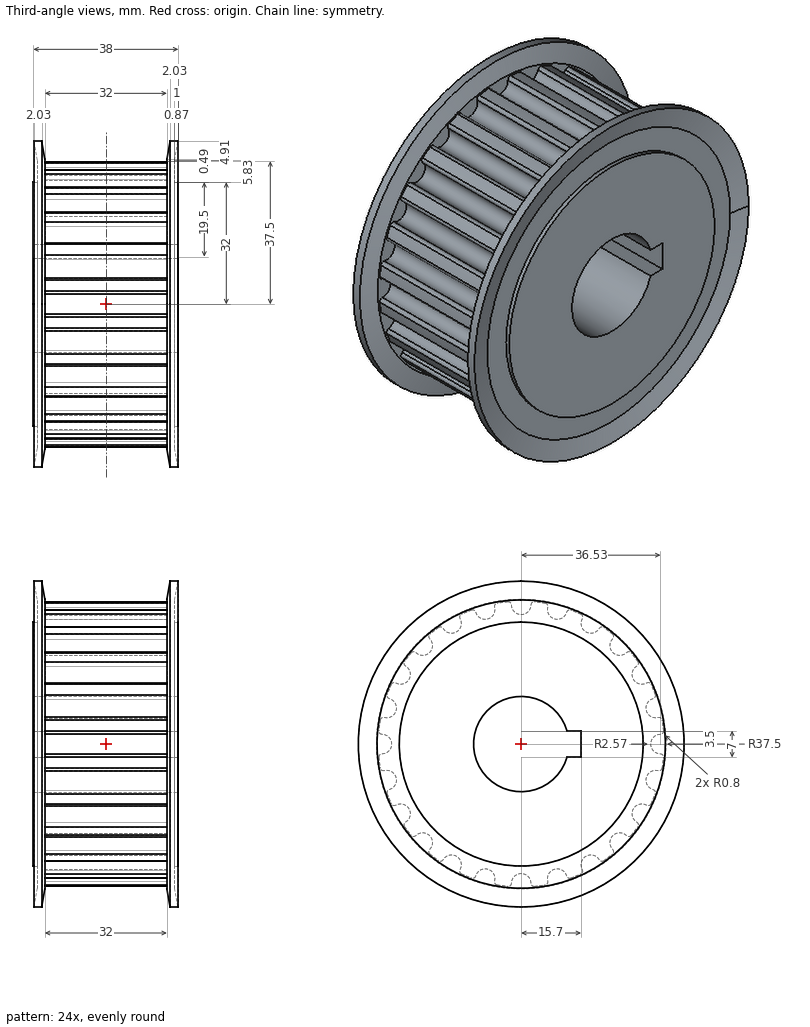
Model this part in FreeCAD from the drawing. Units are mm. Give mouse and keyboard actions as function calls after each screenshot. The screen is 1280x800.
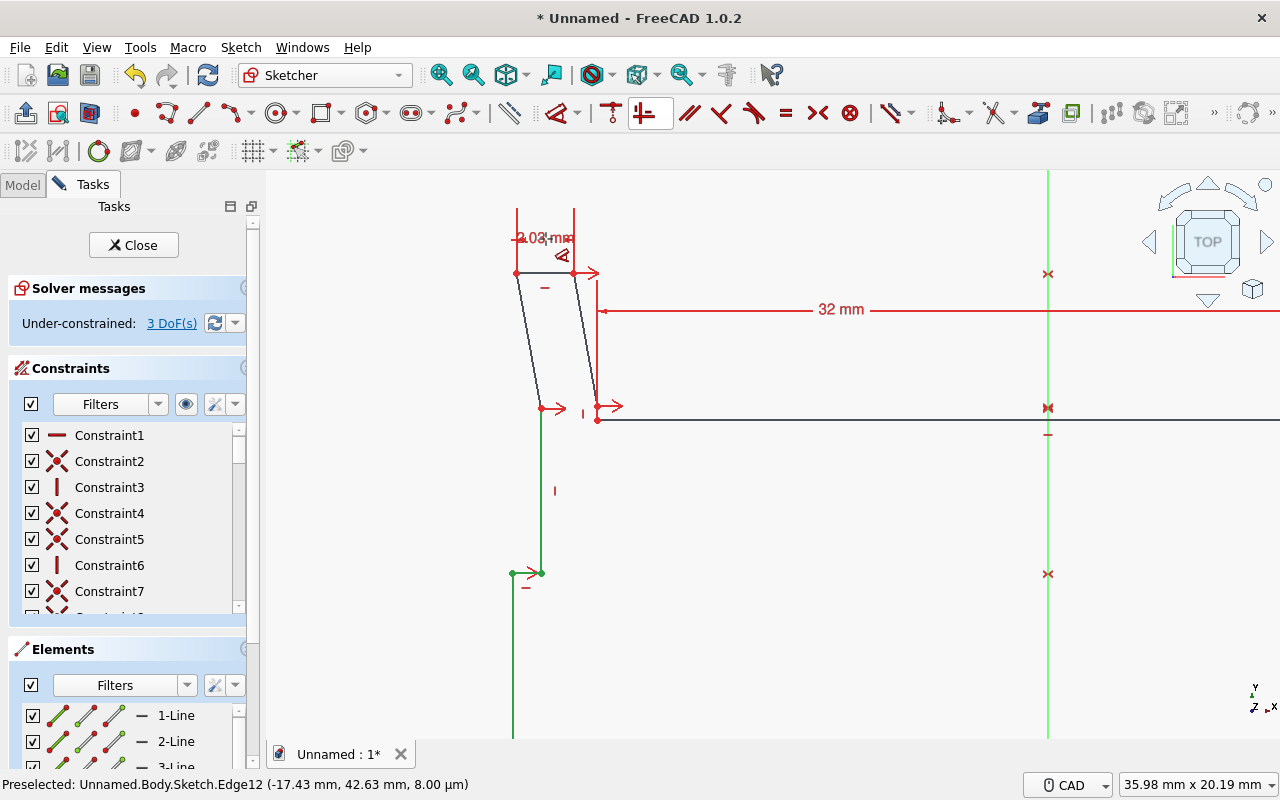
scroll(556, 274, down, 6)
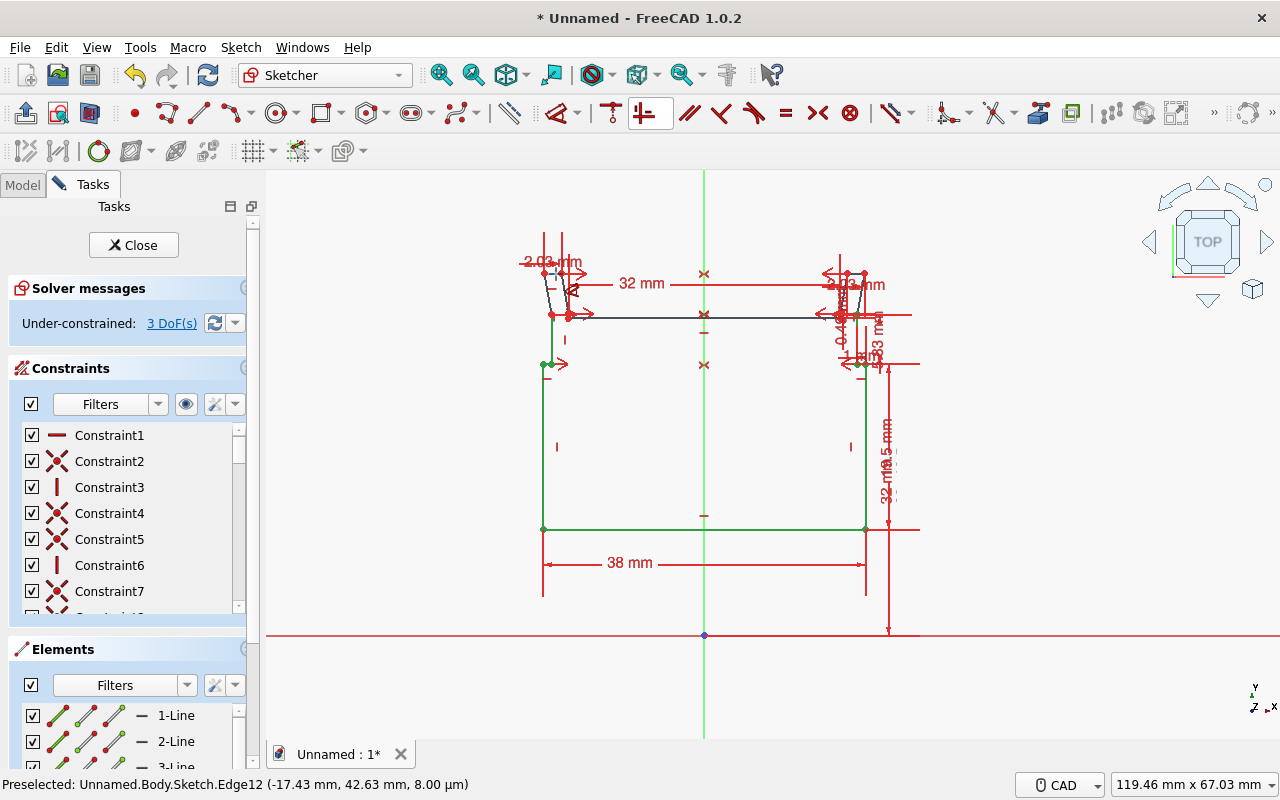
scroll(840, 318, up, 6)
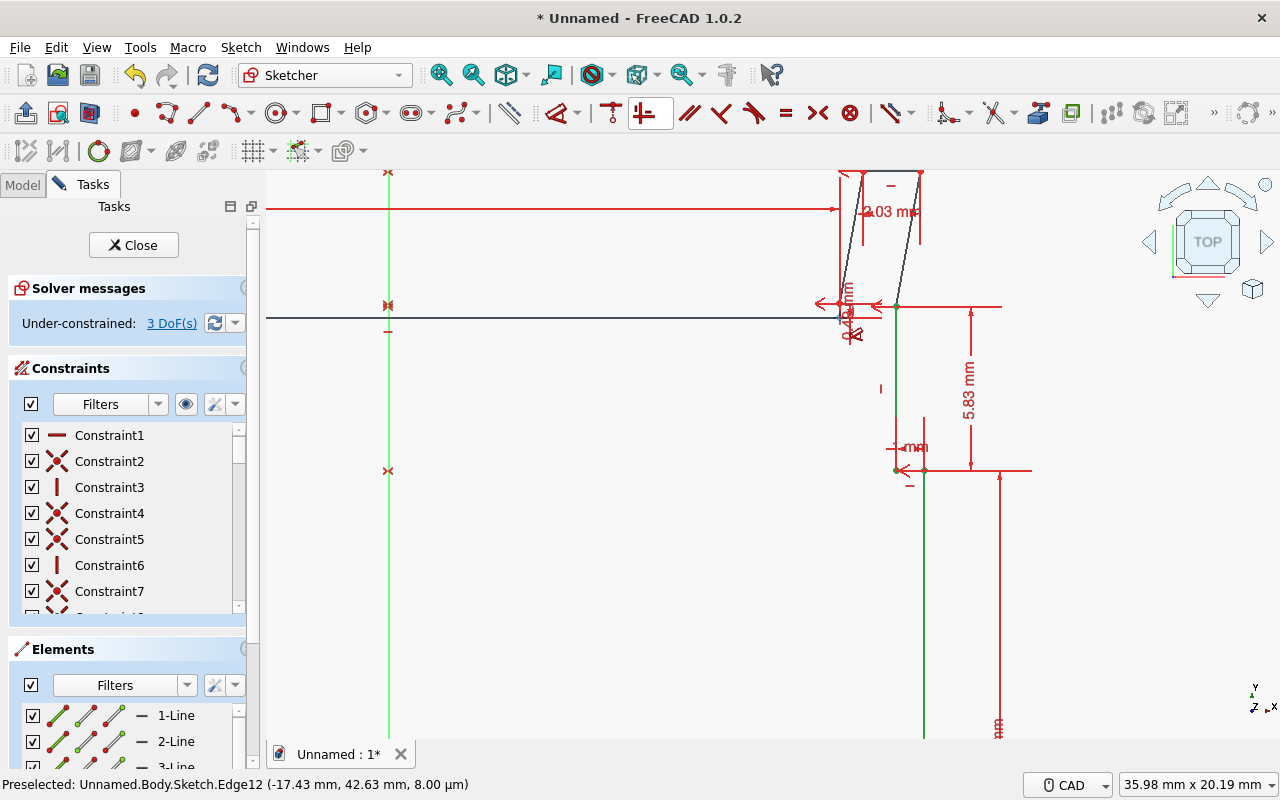
click(840, 318)
click(874, 514)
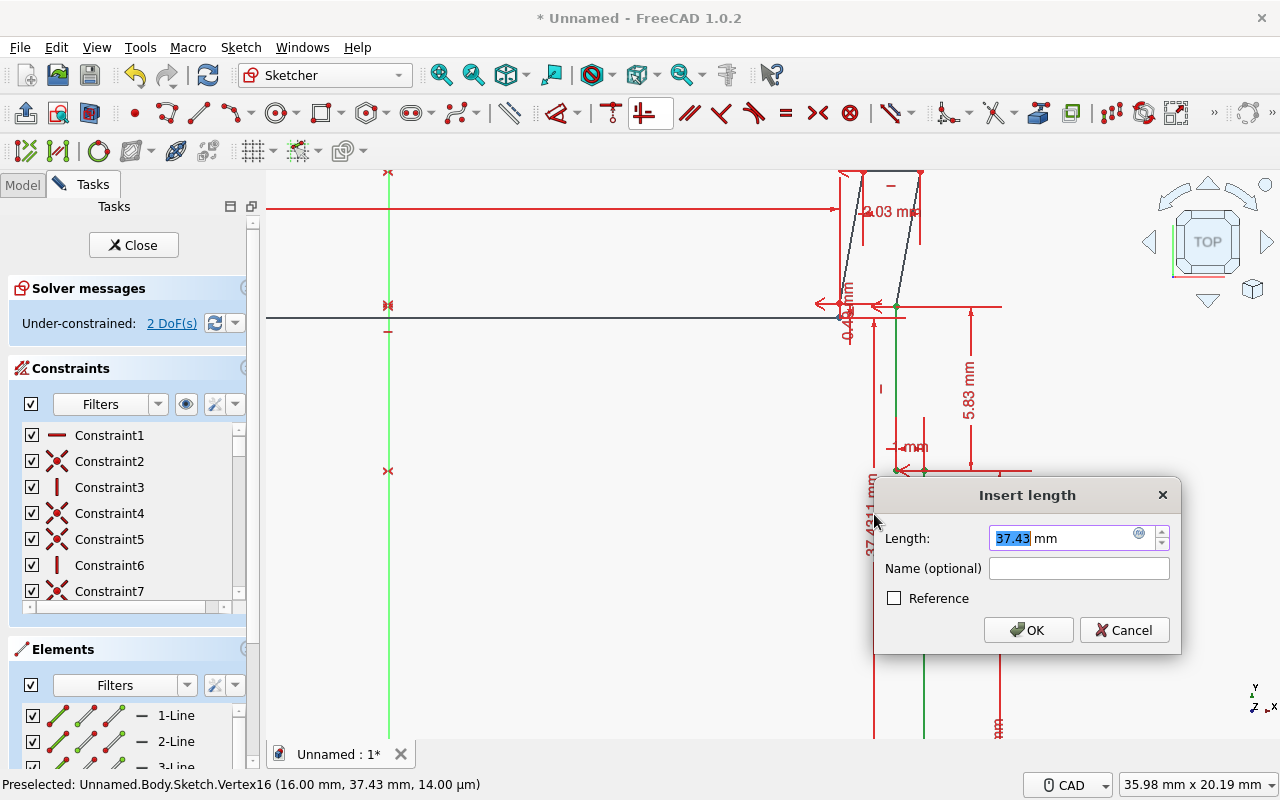
text(37.5)
key(Return)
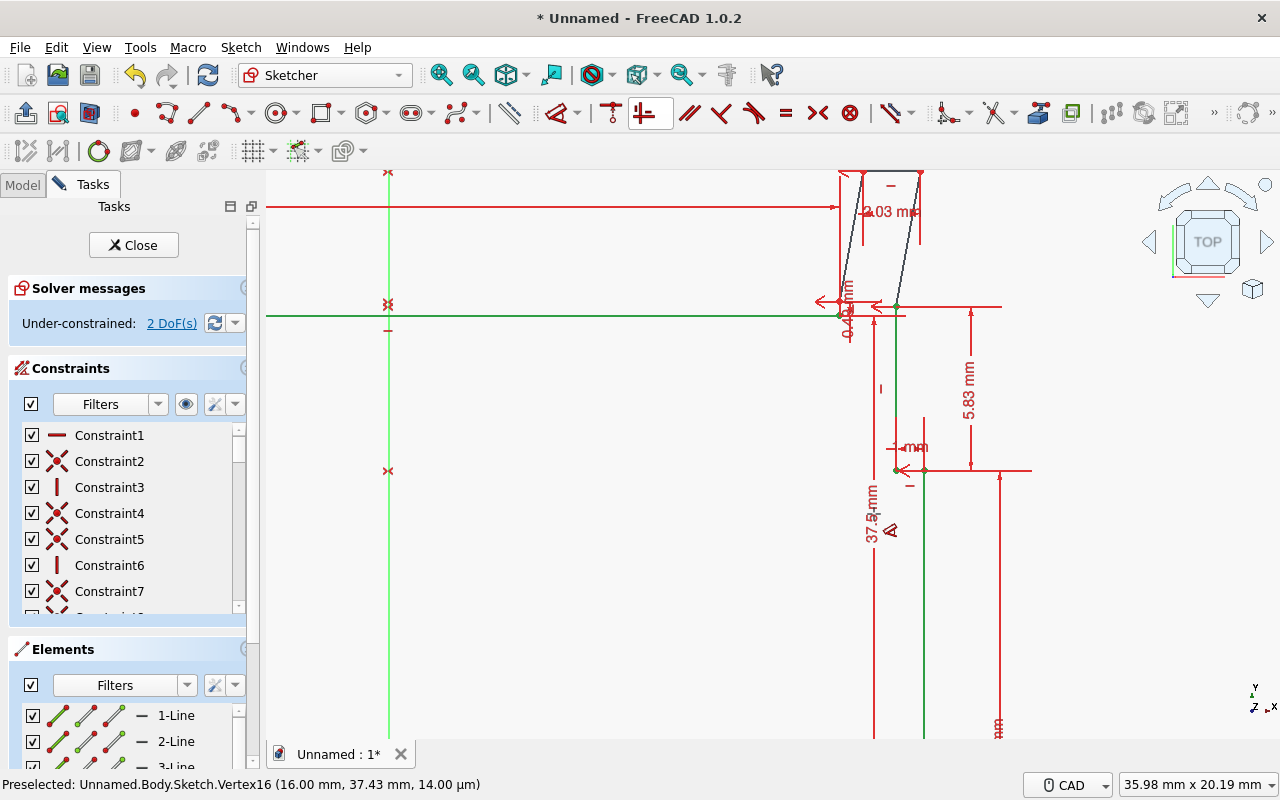
scroll(903, 266, up, 3)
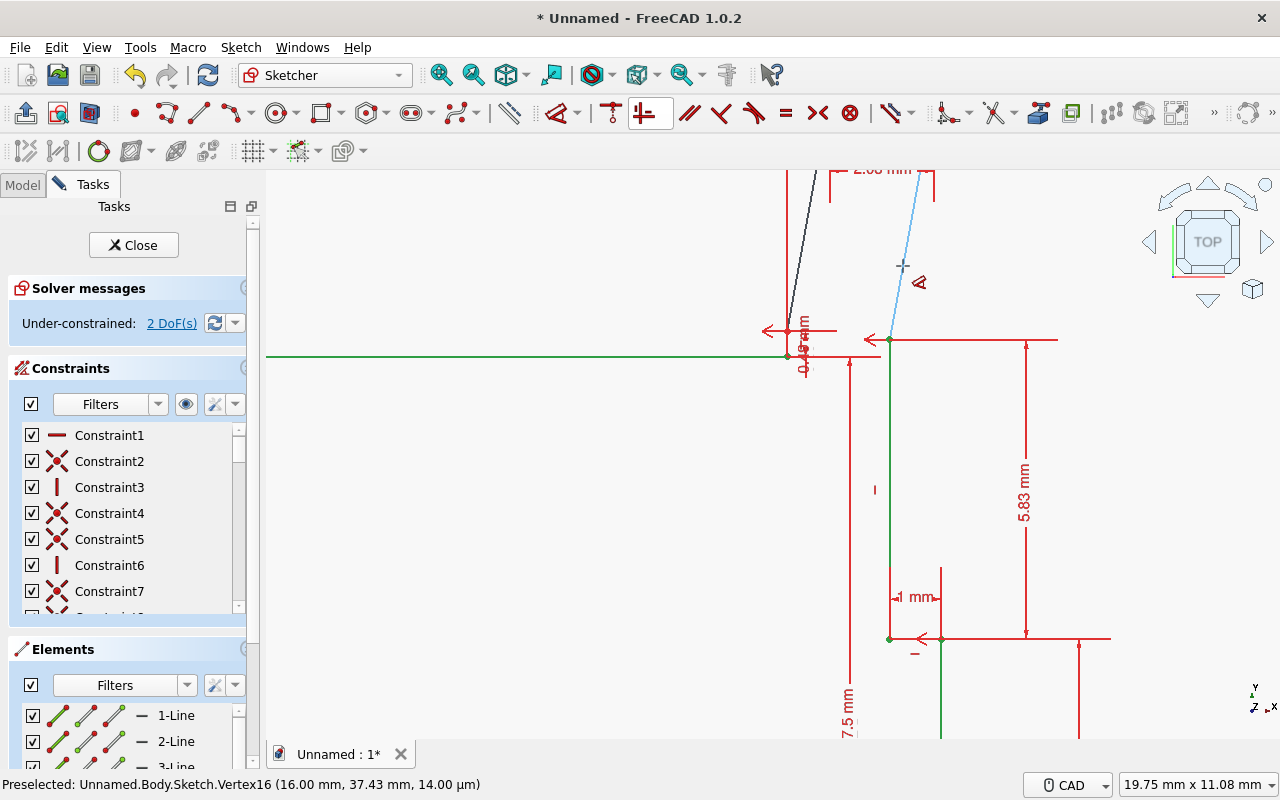
click(903, 266)
click(912, 374)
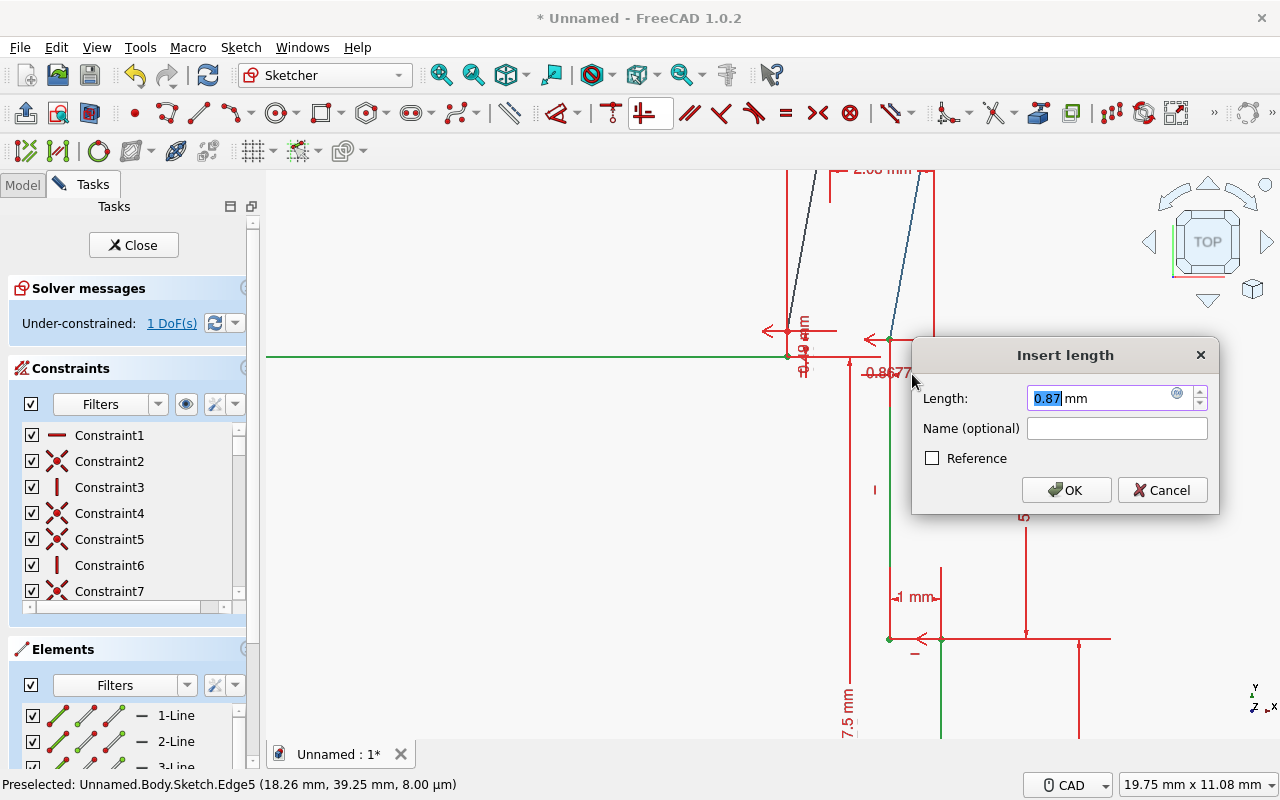
text(0.87)
key(Return)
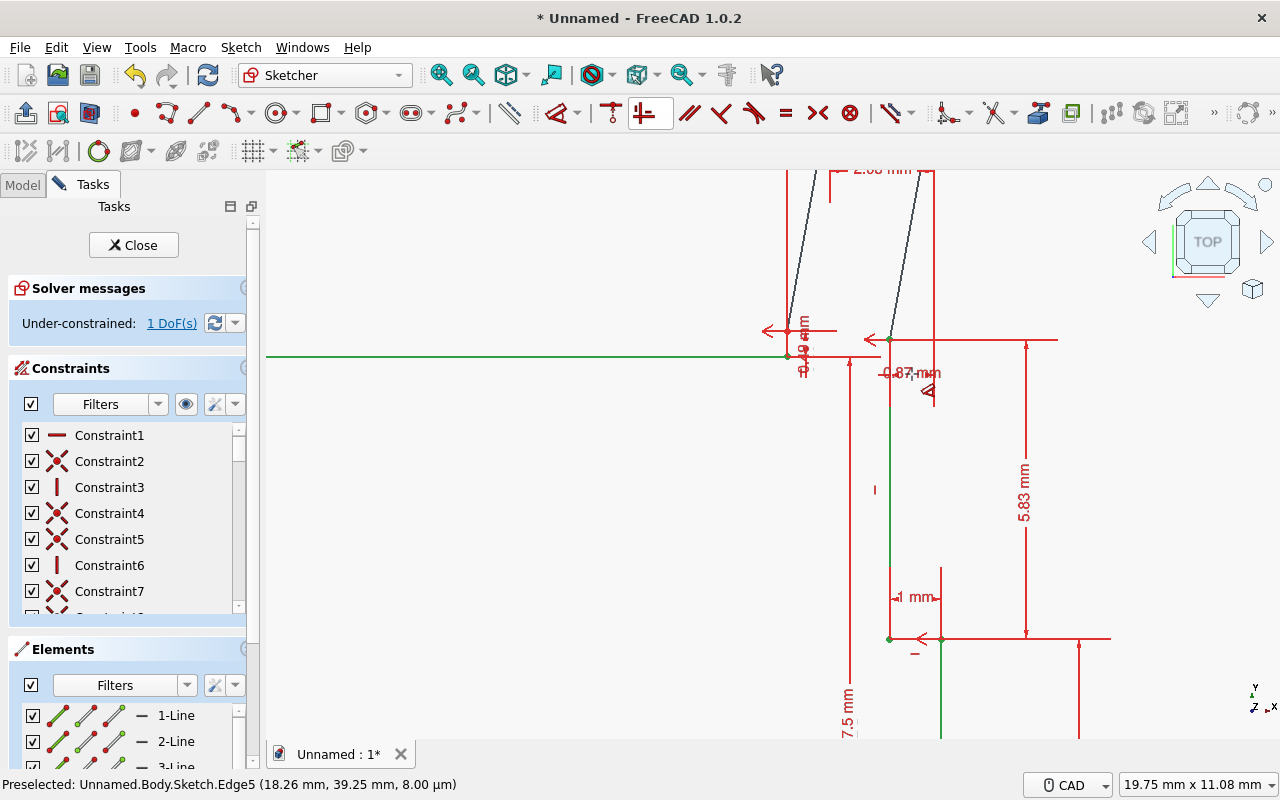
scroll(851, 310, down, 9)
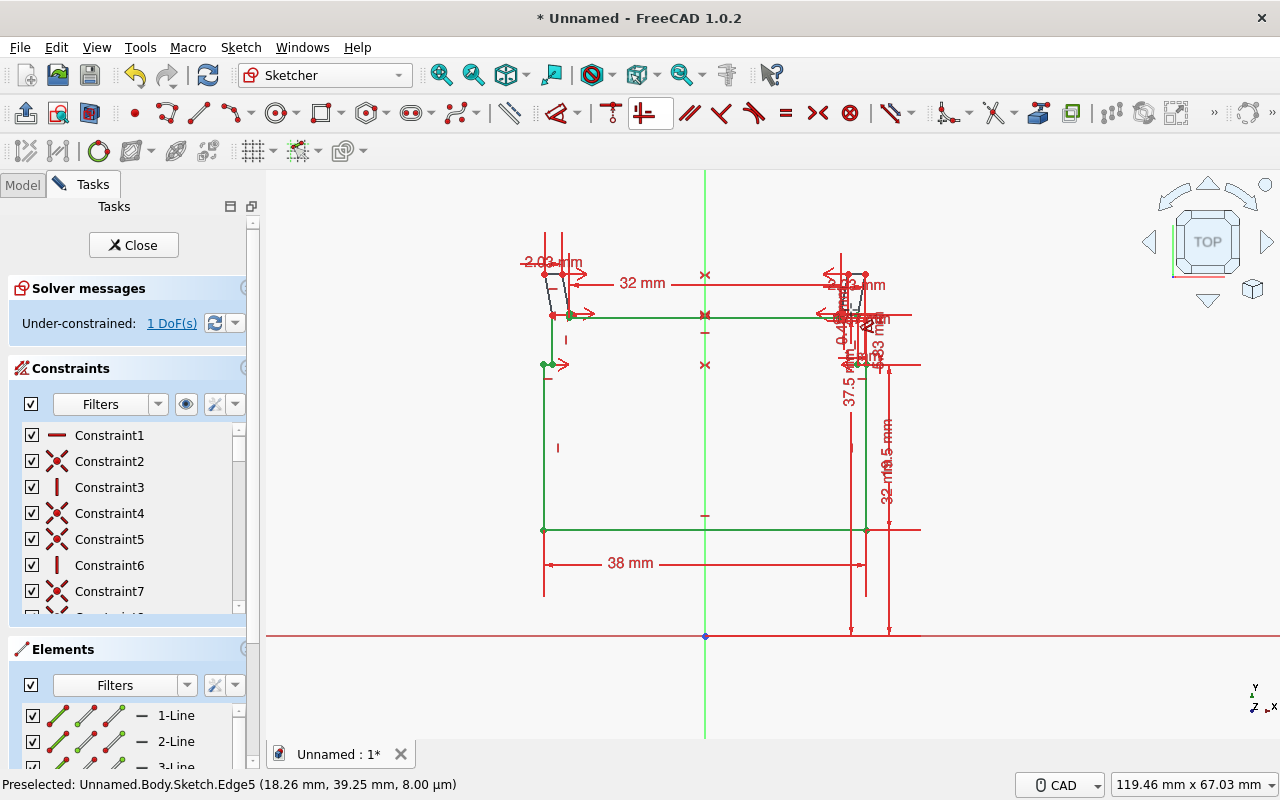
click(860, 303)
click(947, 295)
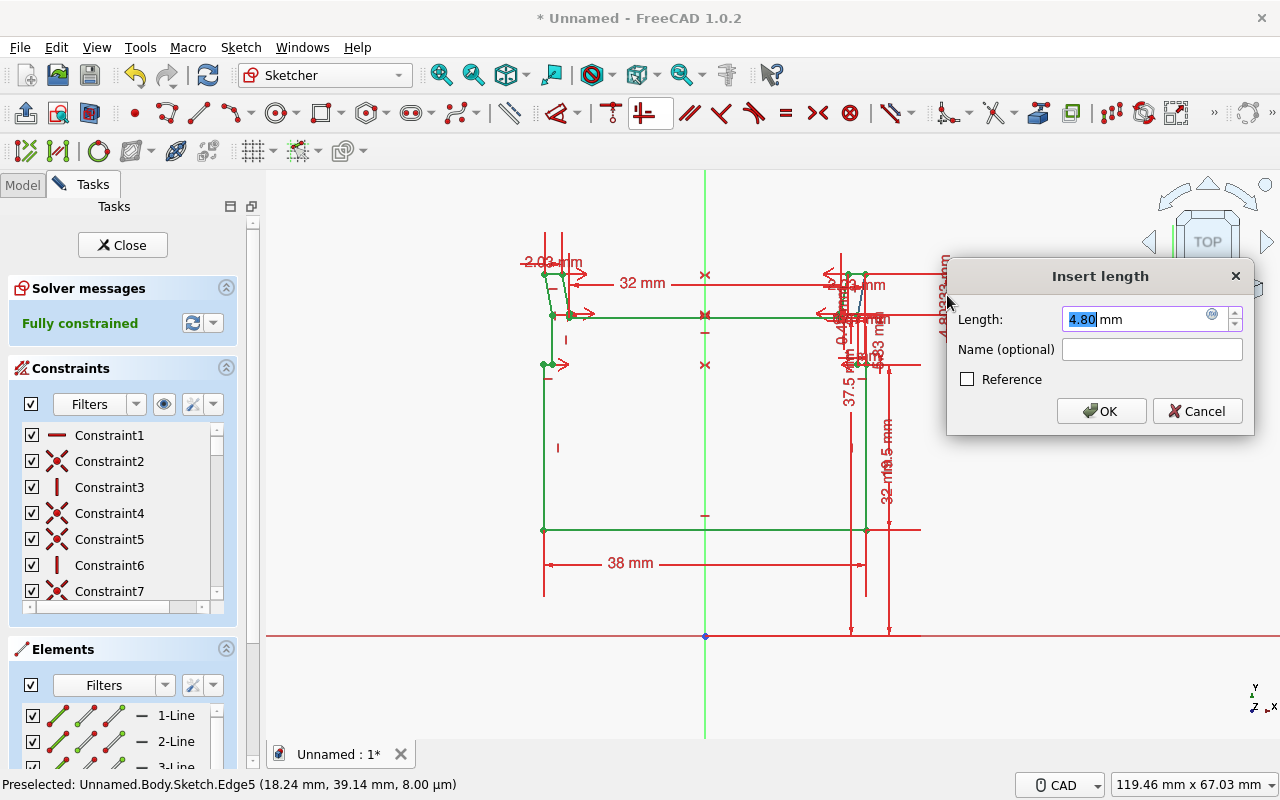
text(4.91)
key(Return)
key(Escape)